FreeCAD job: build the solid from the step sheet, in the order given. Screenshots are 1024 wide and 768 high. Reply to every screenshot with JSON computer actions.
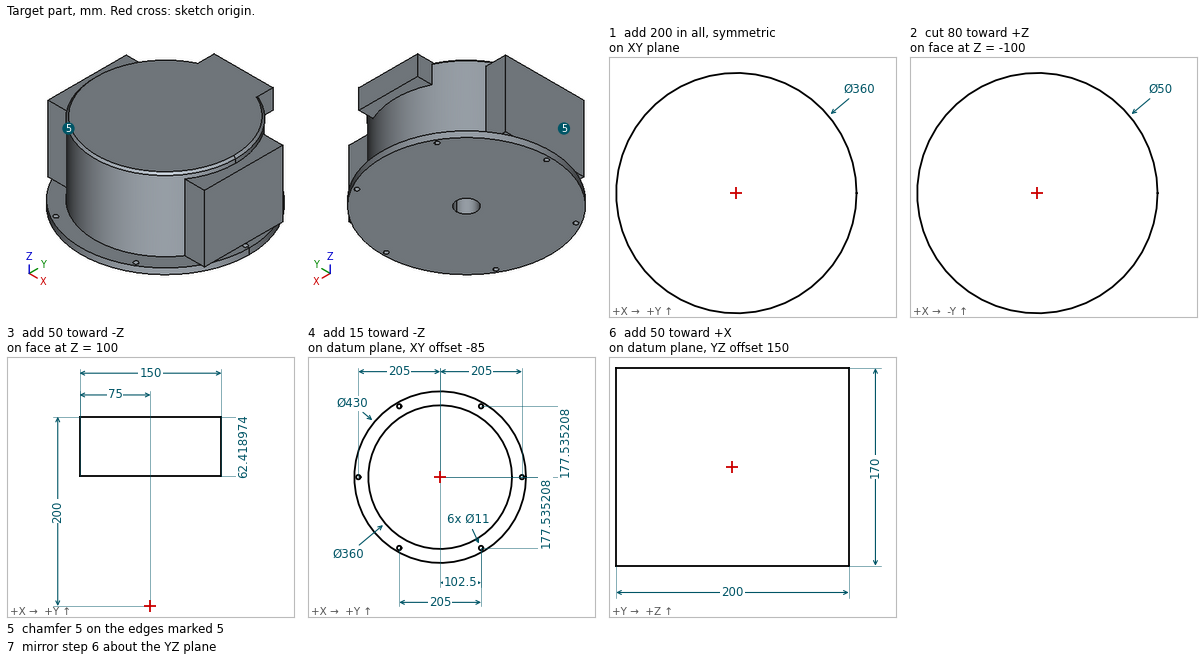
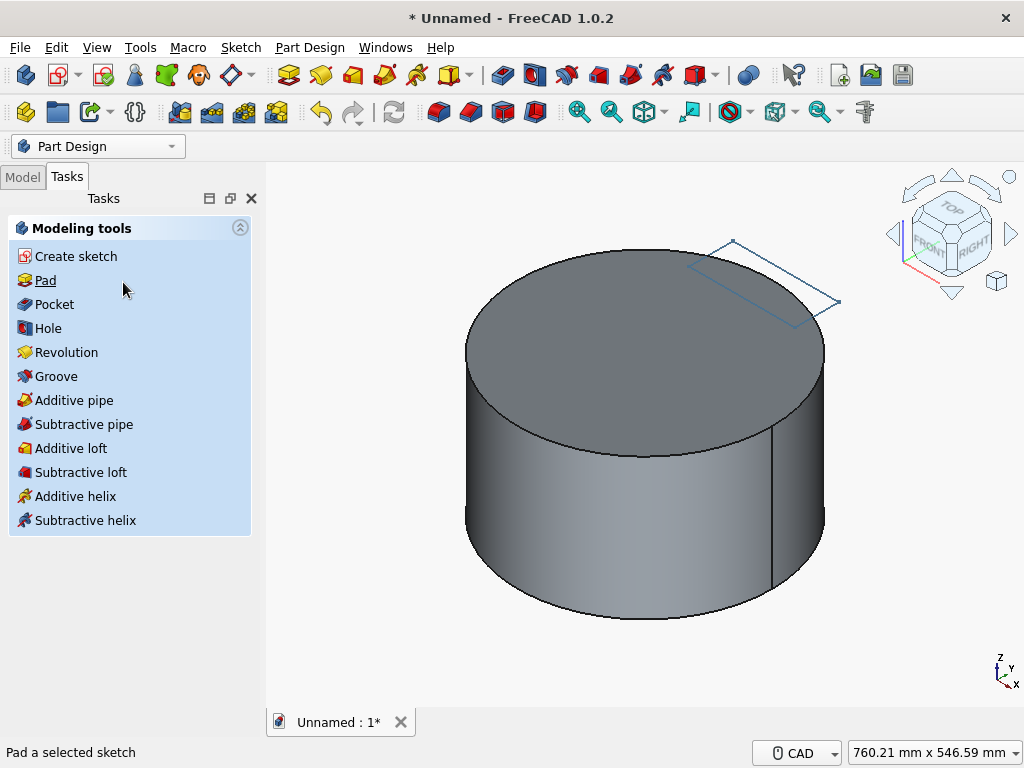
{"action": "left_click", "coordinate": [290, 76]}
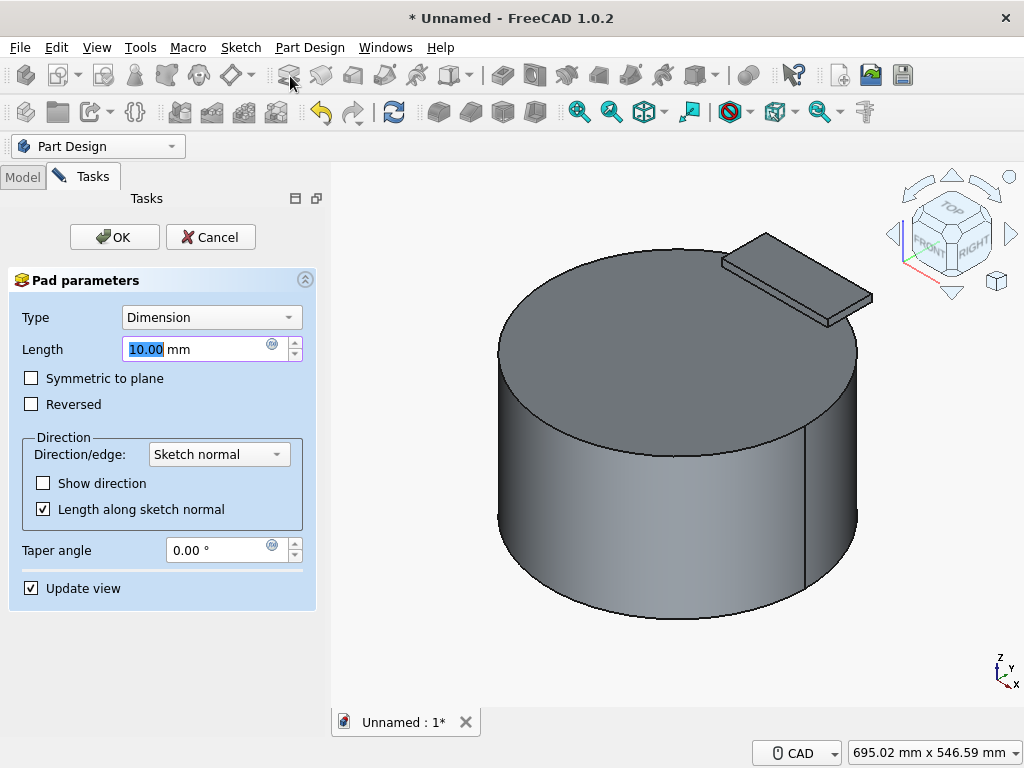
{"action": "type", "text": "50"}
{"action": "key", "text": "Tab"}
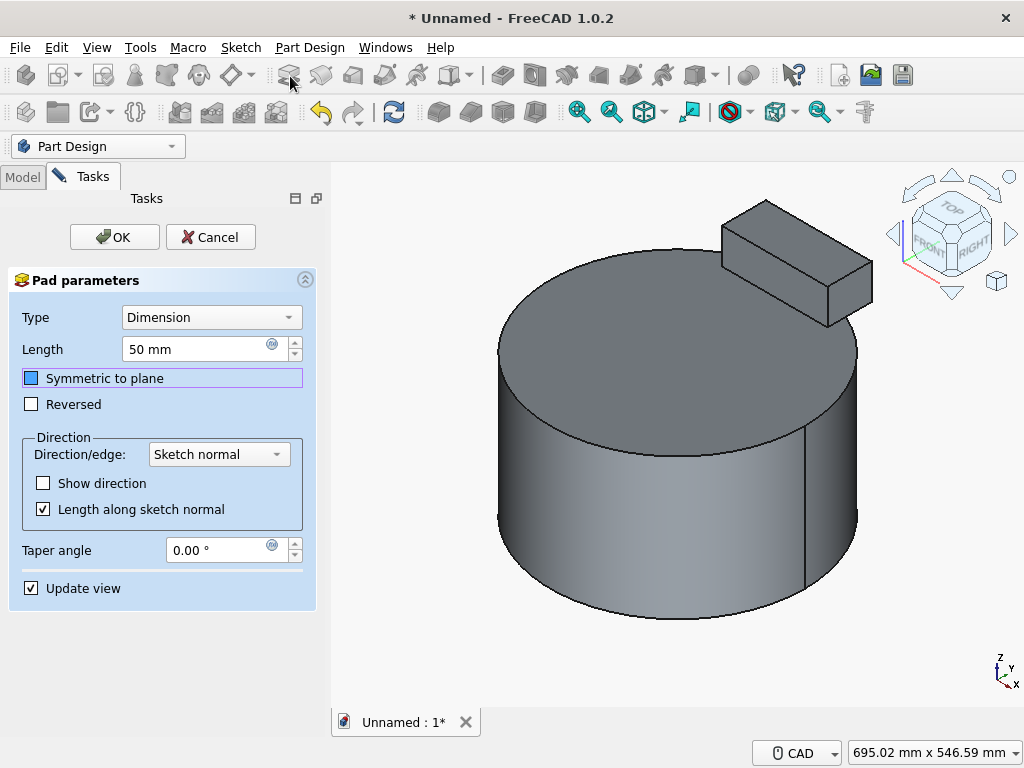
{"action": "left_click", "coordinate": [30, 404]}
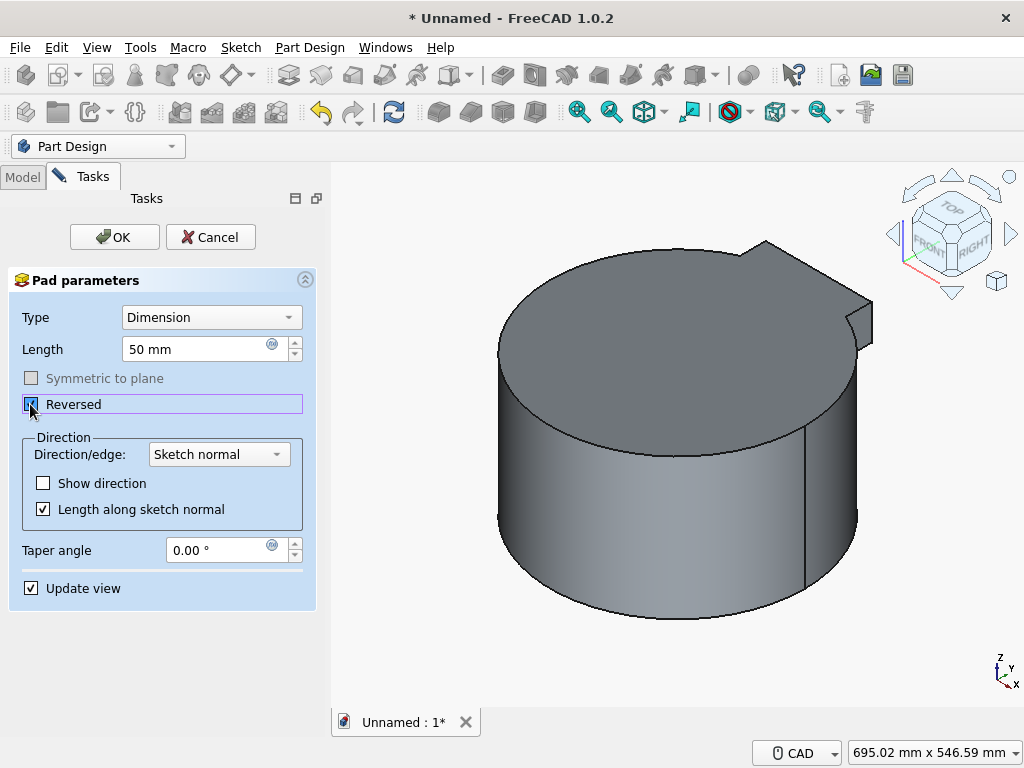
{"action": "left_click", "coordinate": [115, 237]}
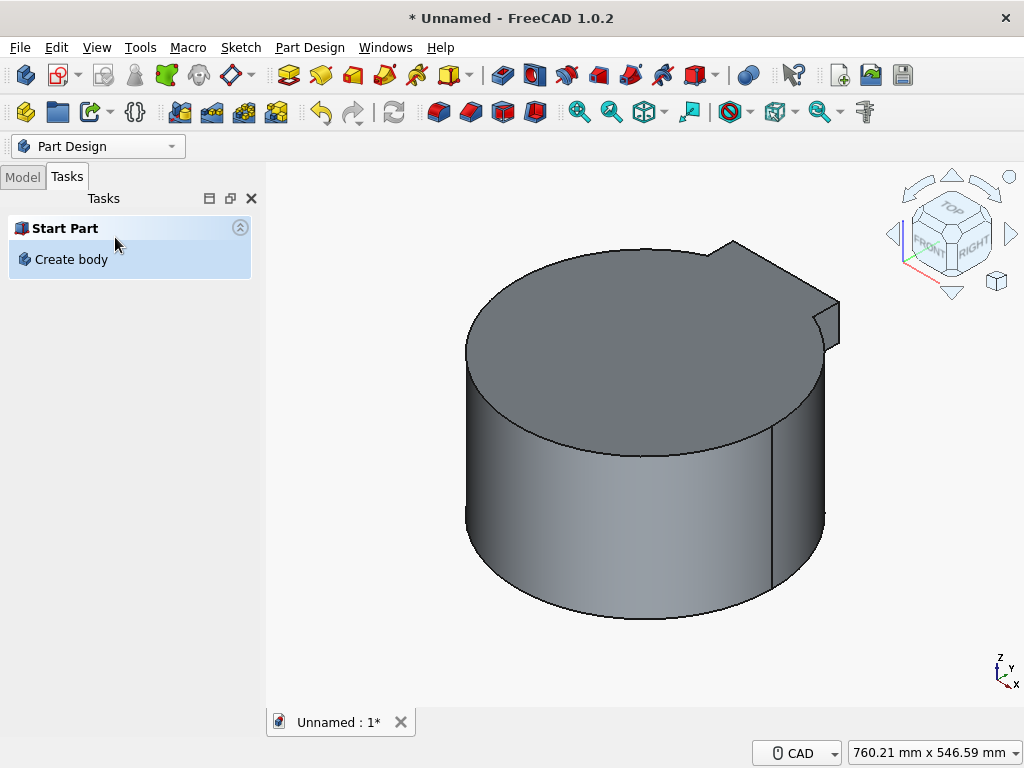
{"action": "left_click", "coordinate": [23, 176]}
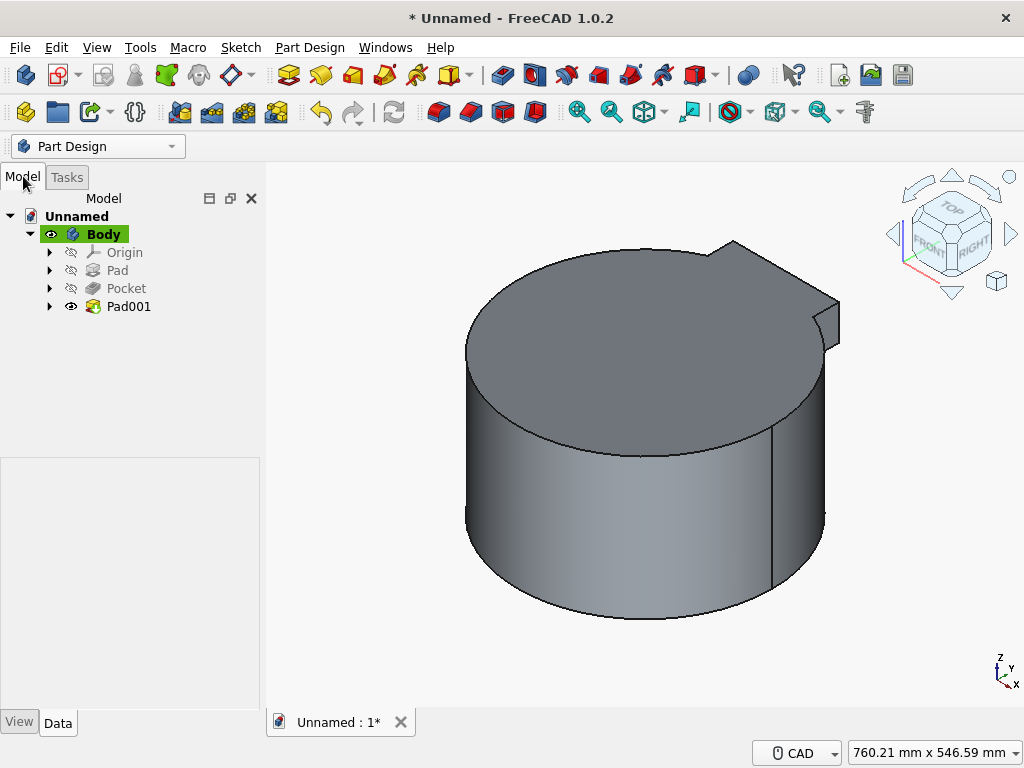
{"action": "left_click", "coordinate": [50, 252]}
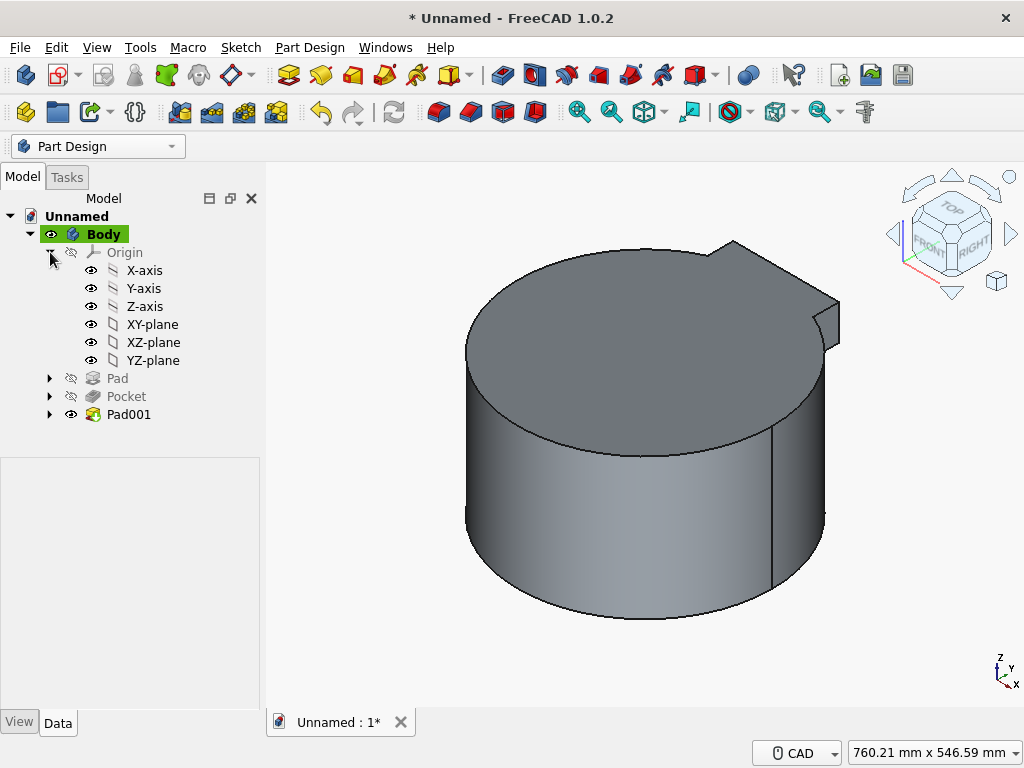
{"action": "left_click", "coordinate": [136, 324]}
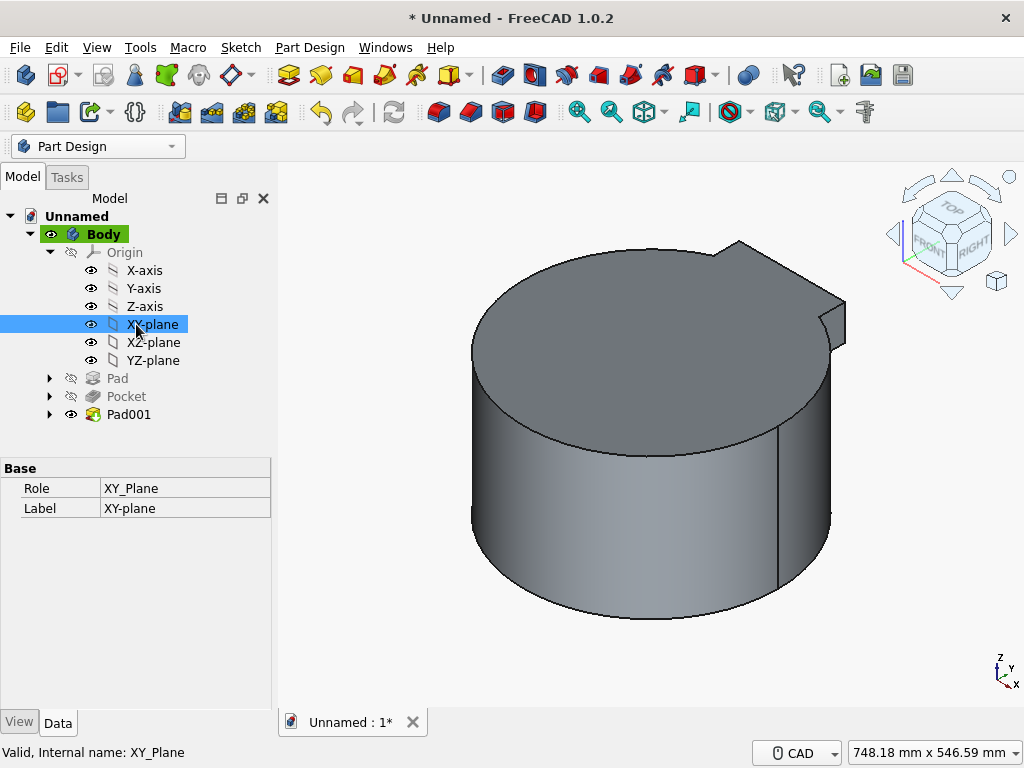
{"action": "left_click", "coordinate": [232, 76]}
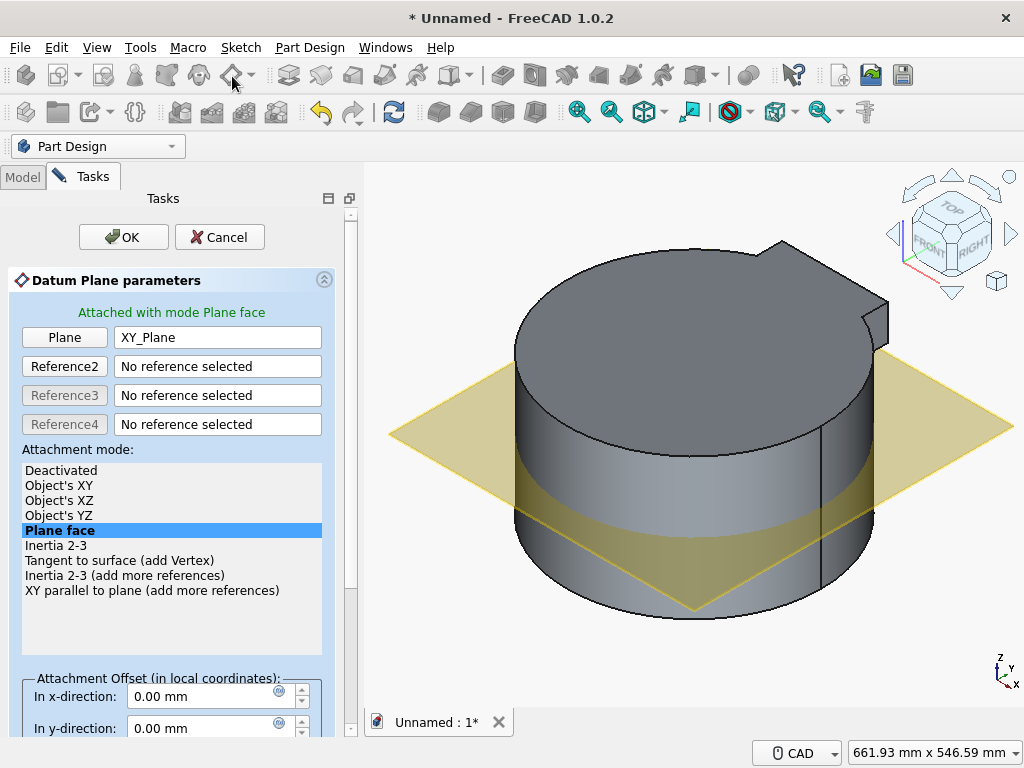
{"action": "scroll", "coordinate": [351, 472], "scroll_direction": "down", "scroll_amount": 2}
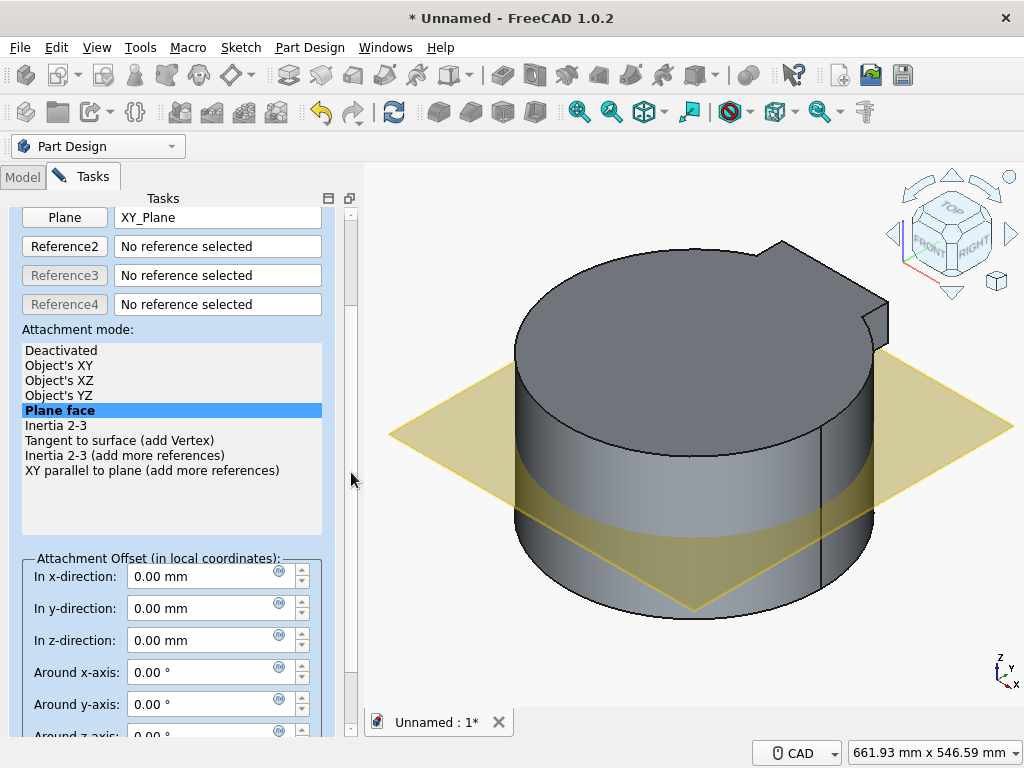
{"action": "triple_click", "coordinate": [210, 640]}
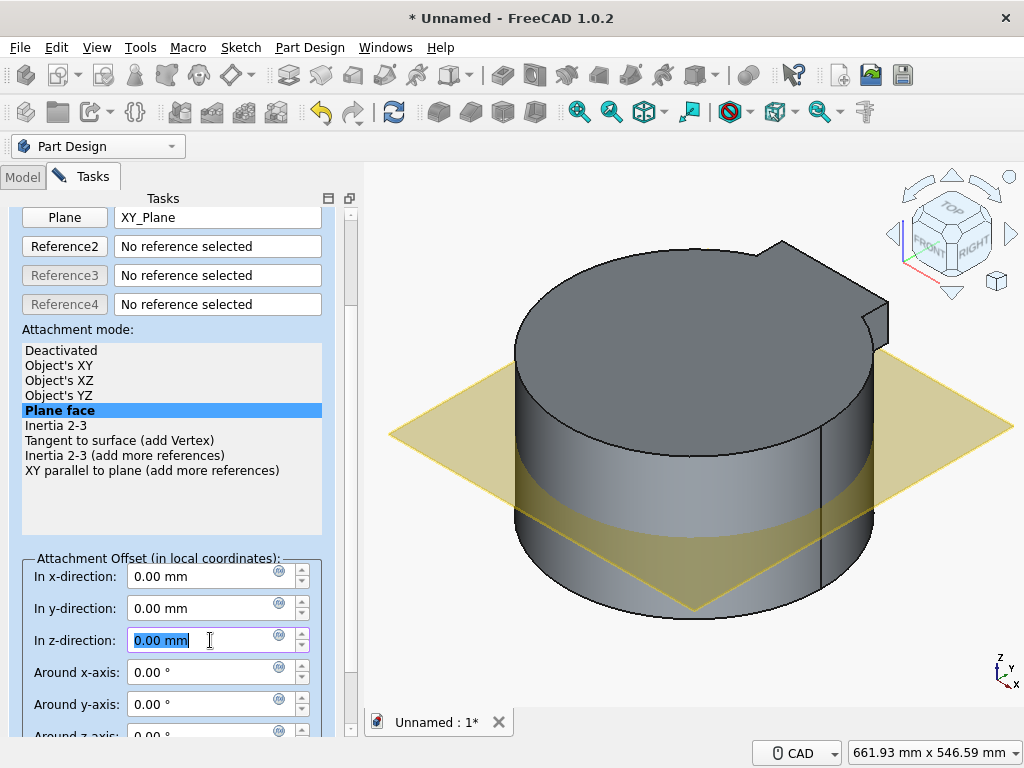
{"action": "type", "text": "-85"}
{"action": "key", "text": "Tab"}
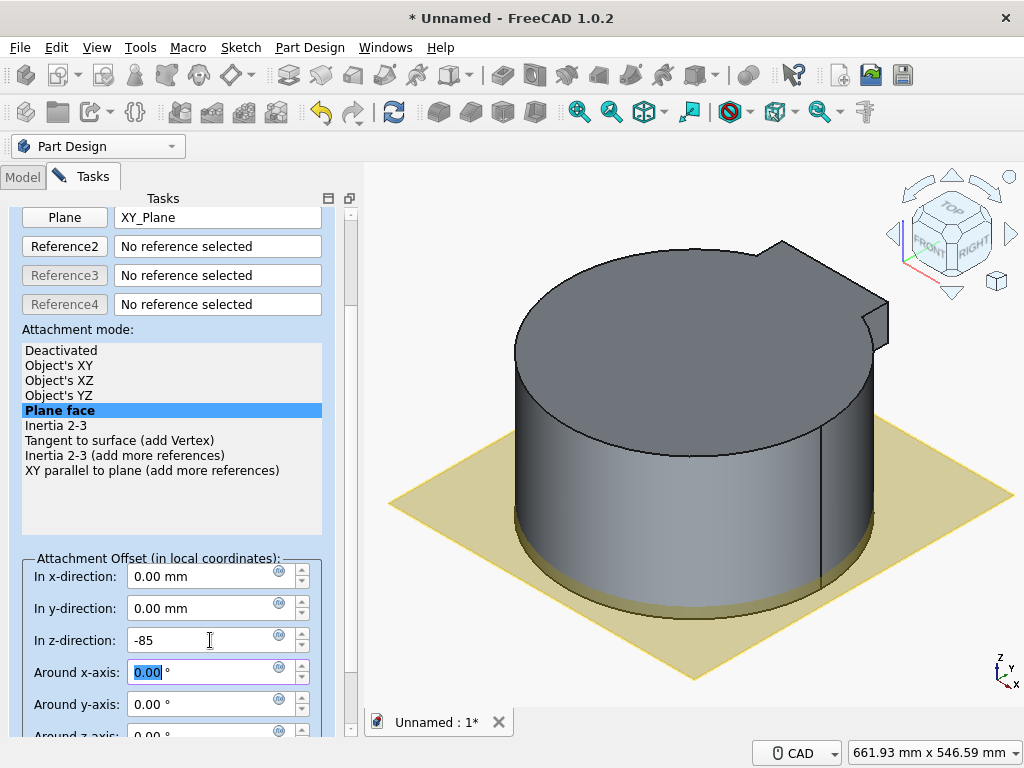
{"action": "scroll", "coordinate": [351, 472], "scroll_direction": "up", "scroll_amount": 3}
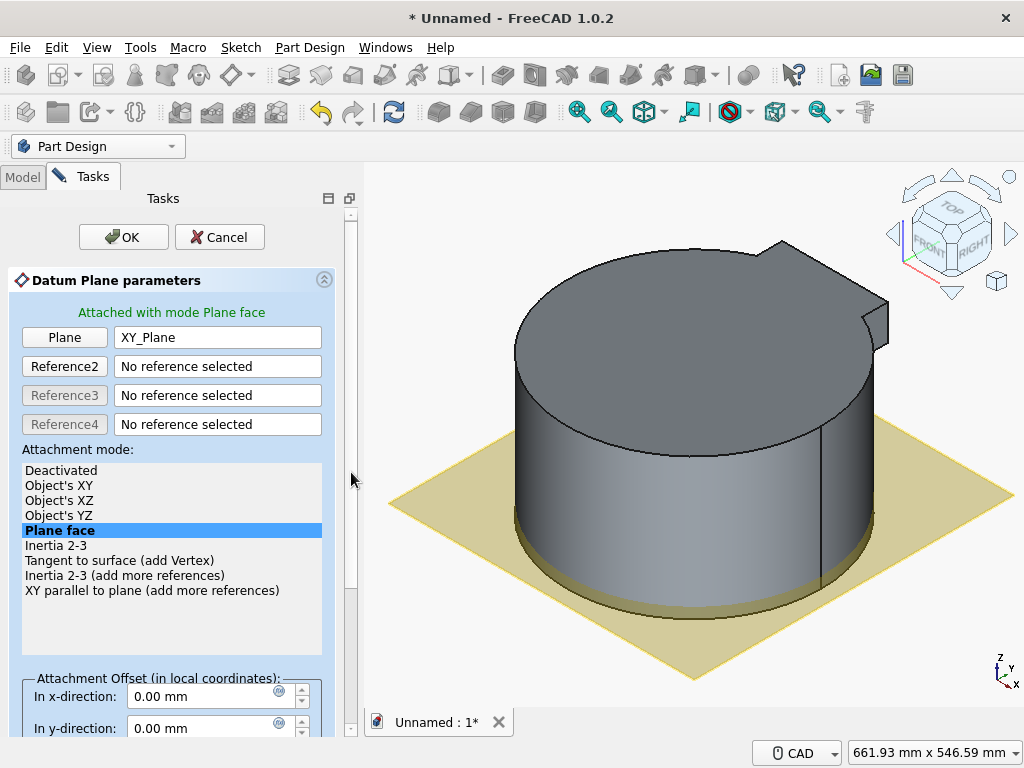
{"action": "left_click", "coordinate": [124, 237]}